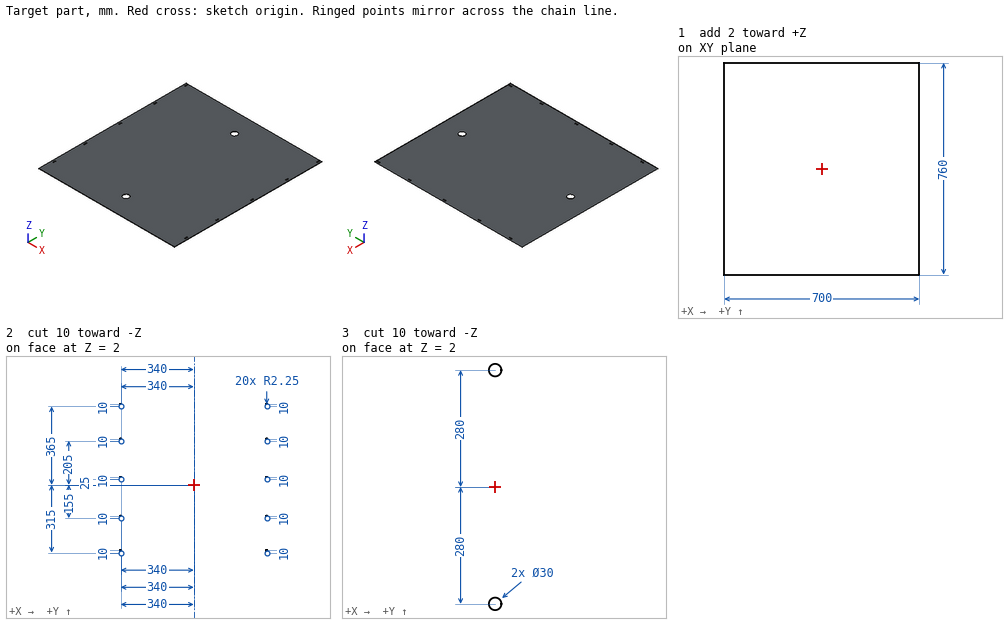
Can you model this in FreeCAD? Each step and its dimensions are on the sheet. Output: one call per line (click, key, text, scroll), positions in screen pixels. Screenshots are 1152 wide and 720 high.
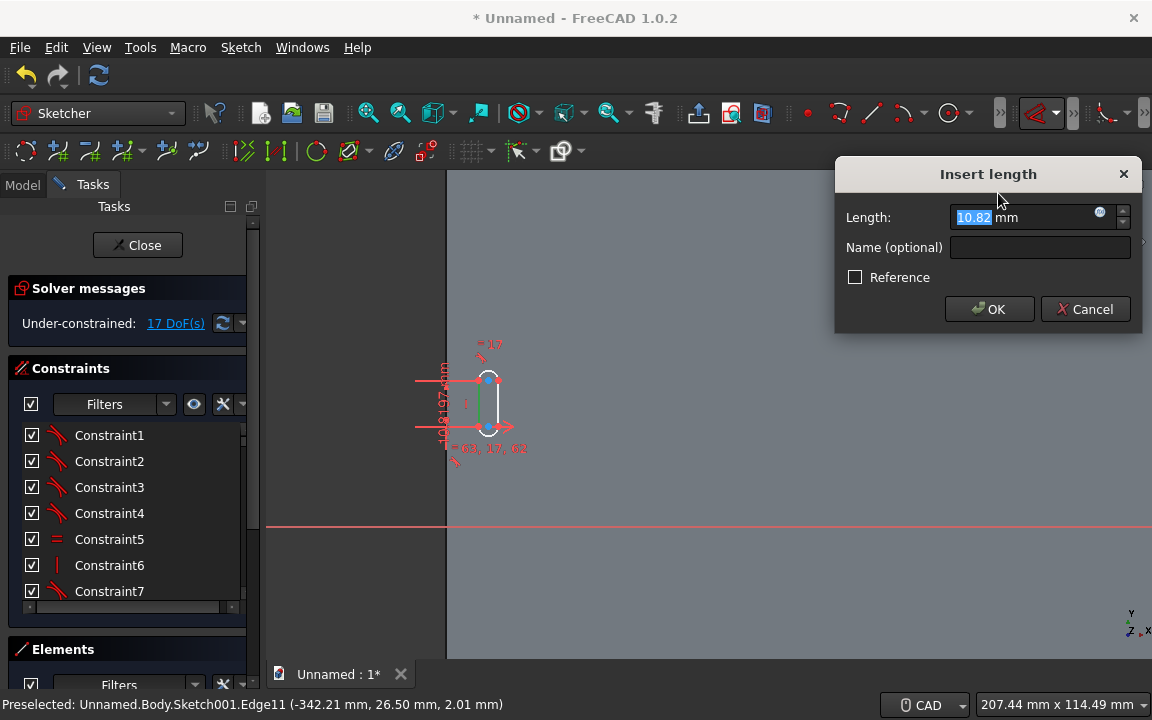
text(10)
key(Return)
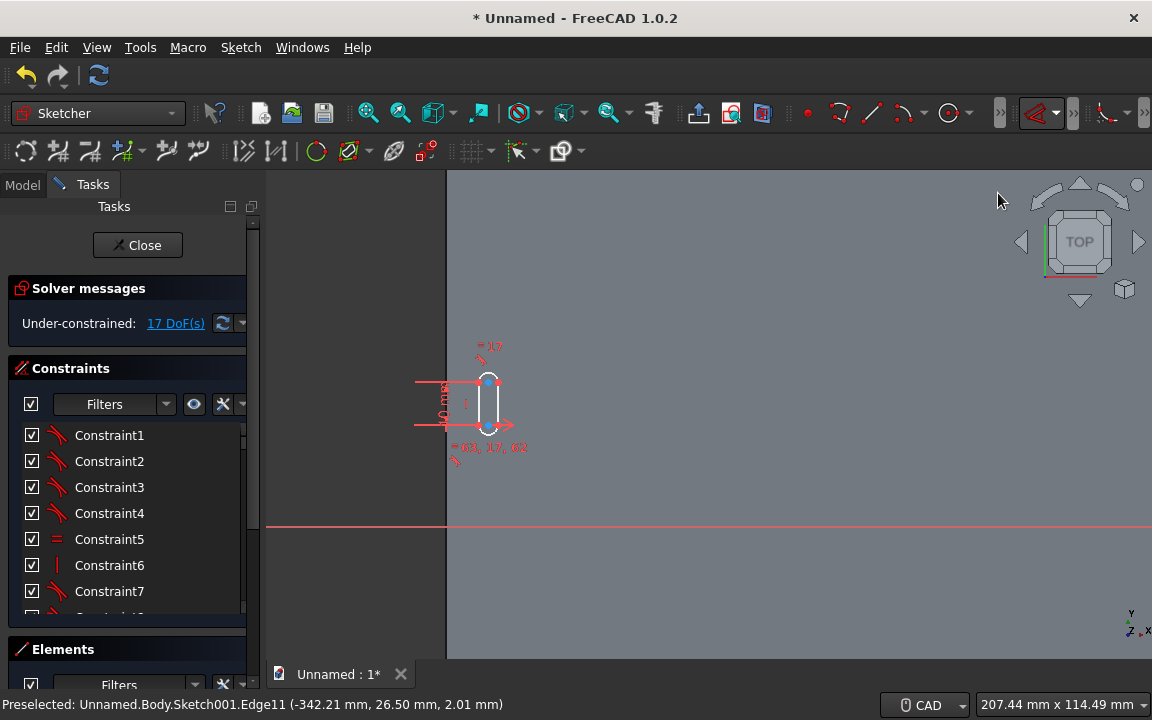
scroll(479, 416, down, 11)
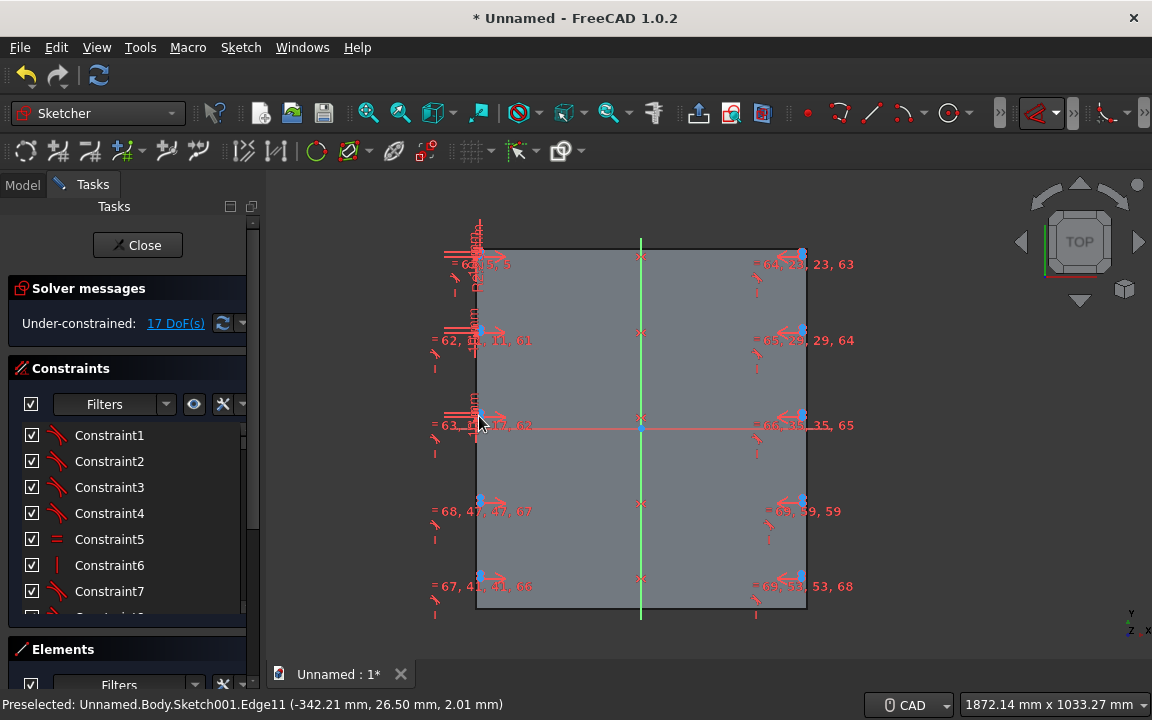
scroll(801, 255, up, 11)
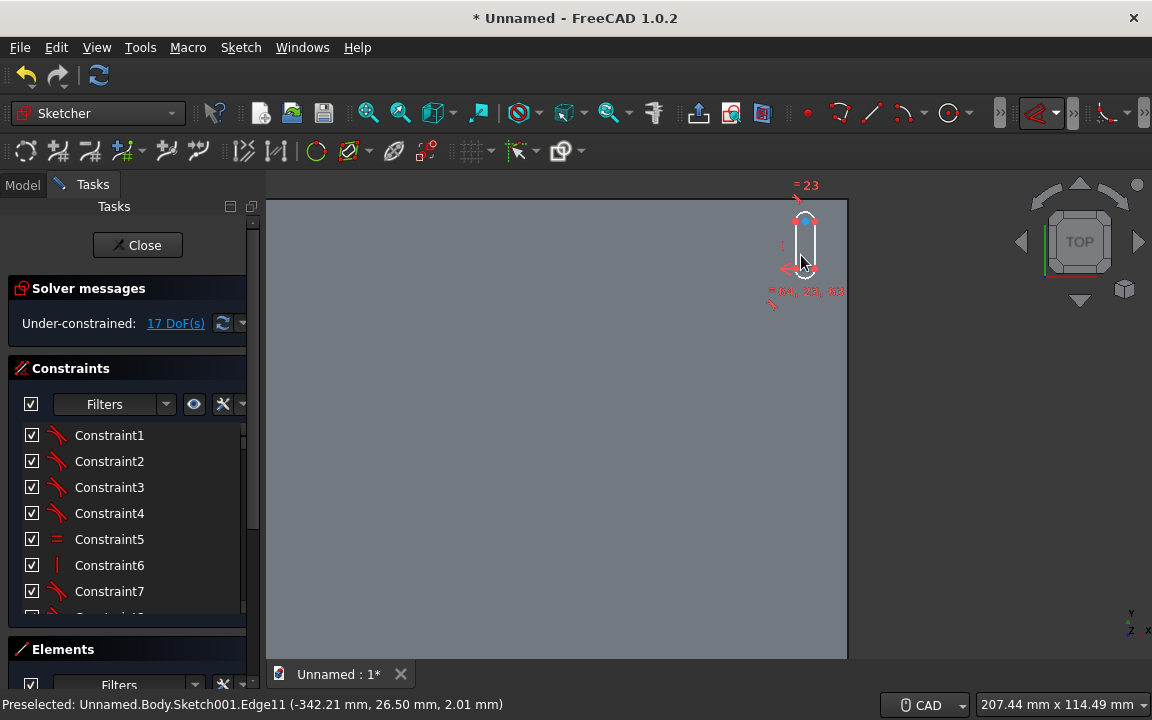
click(796, 255)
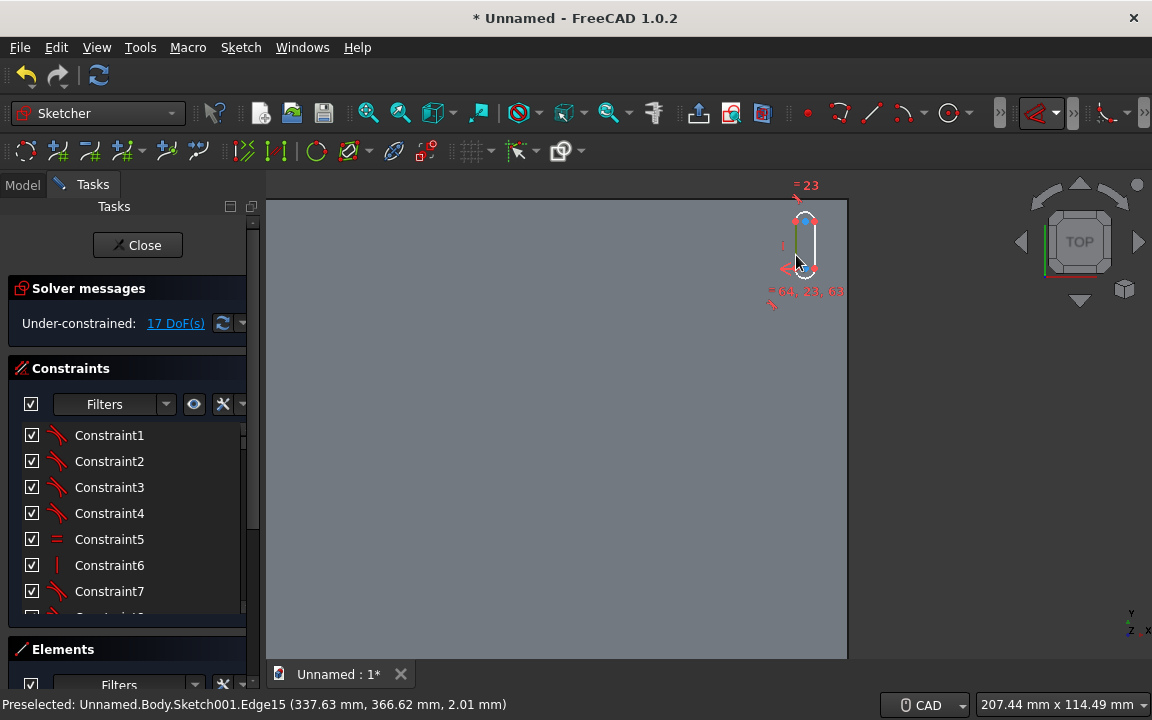
click(1058, 114)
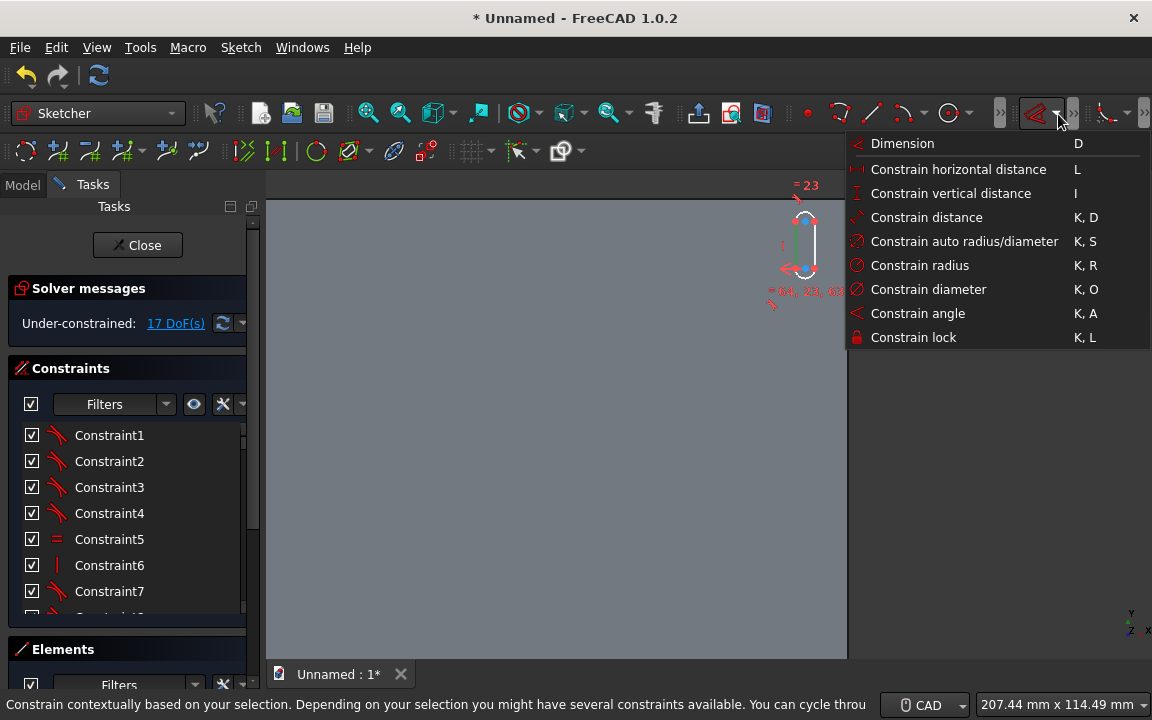
click(998, 193)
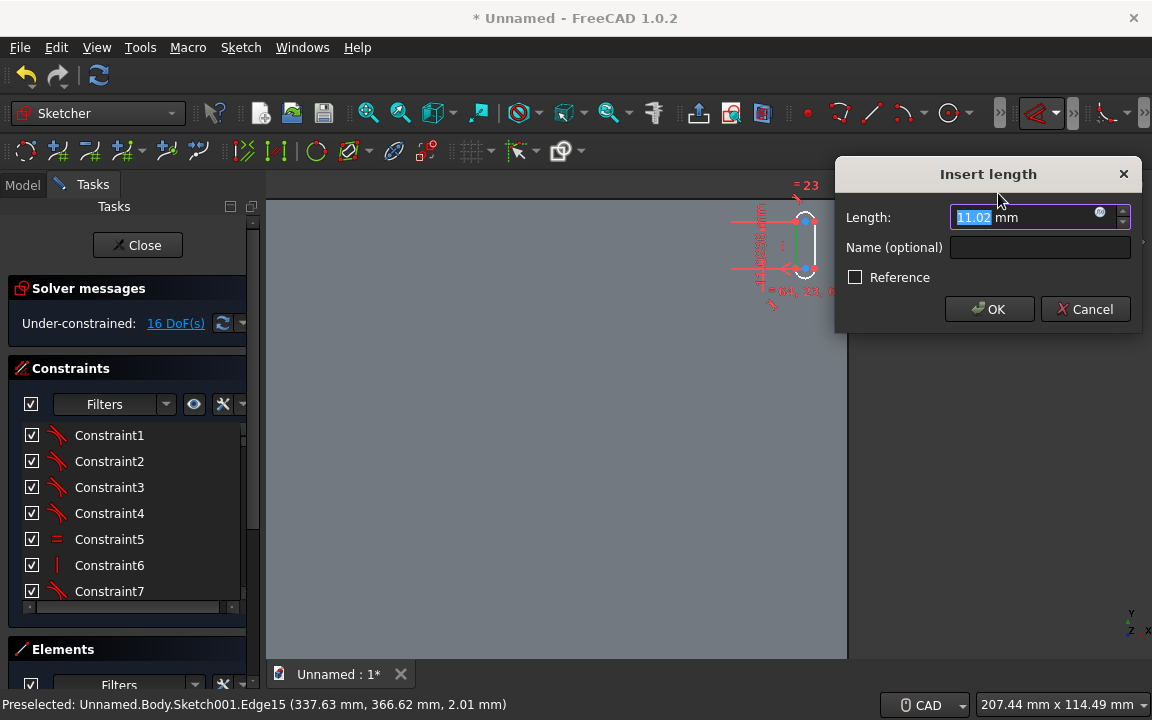
text(10)
key(Return)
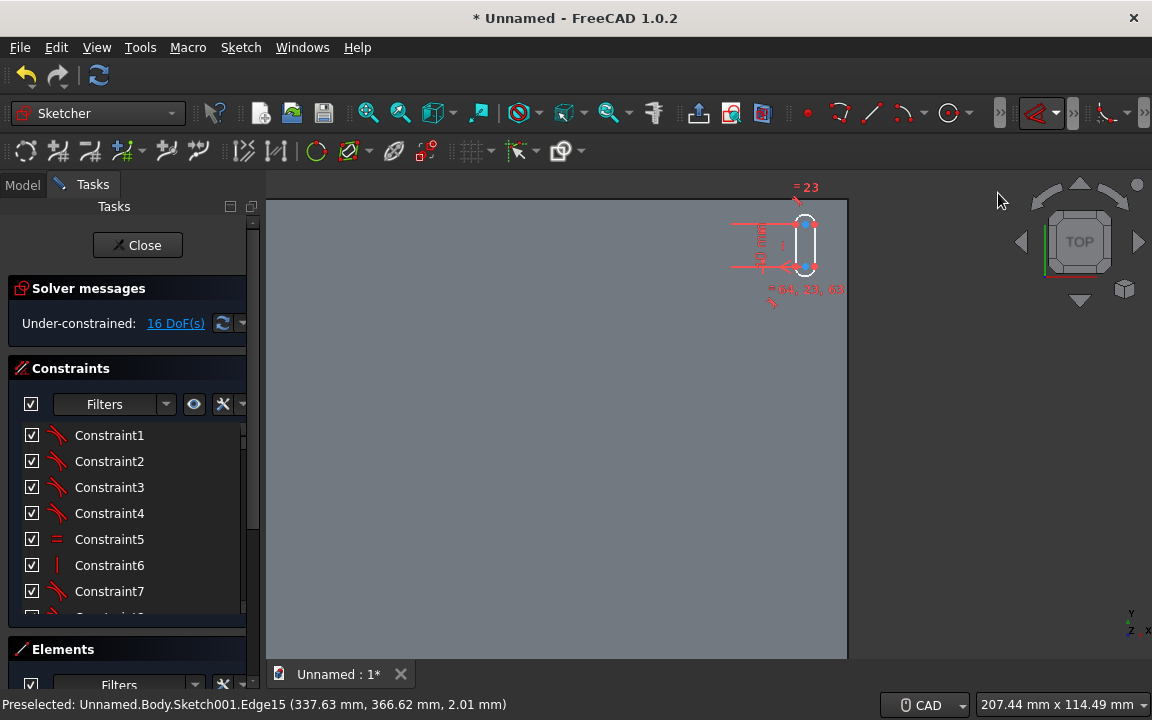
scroll(801, 255, down, 11)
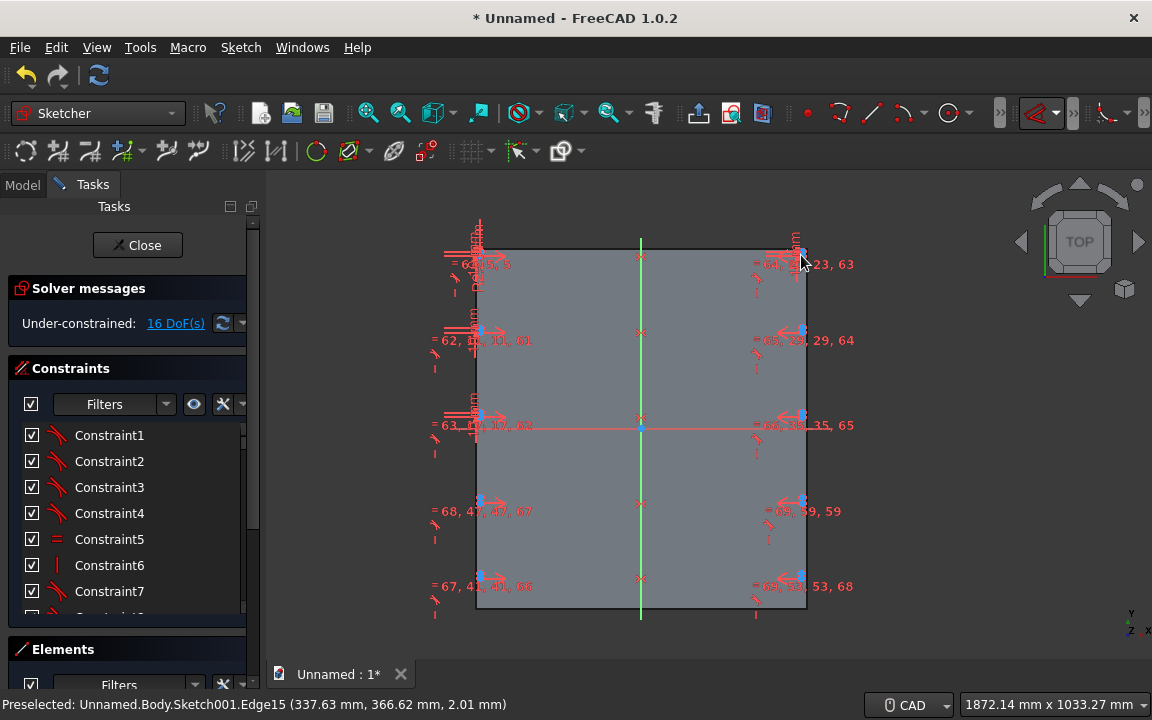
scroll(801, 331, up, 11)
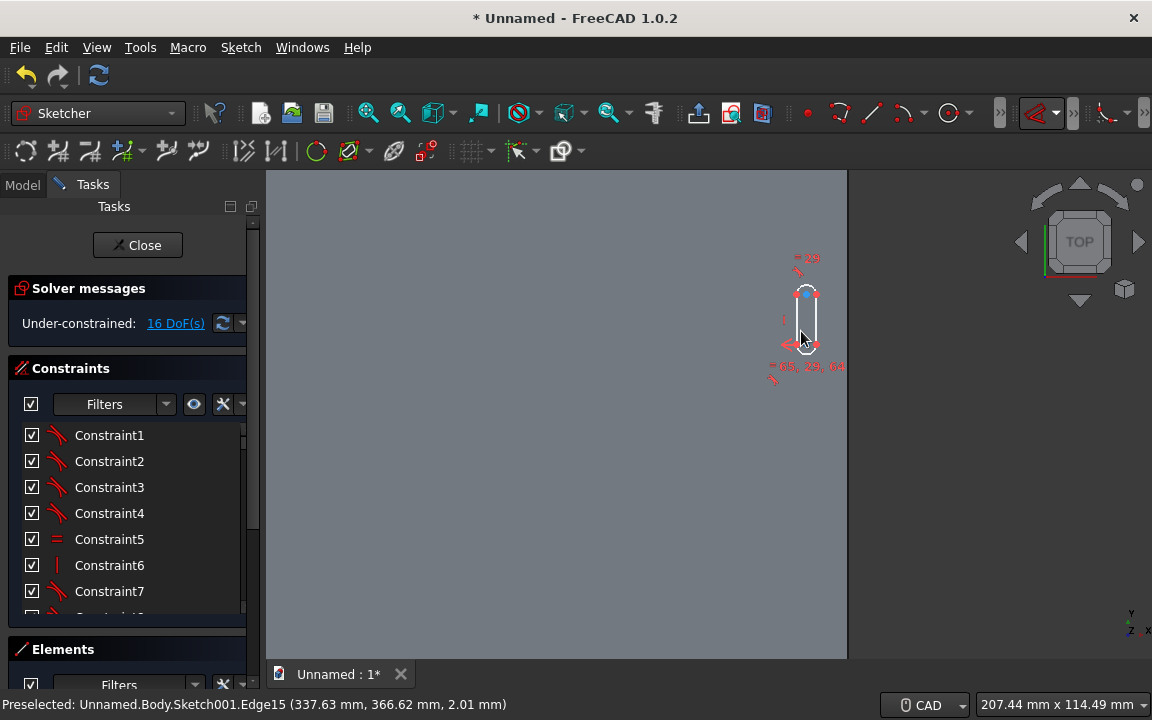
click(797, 330)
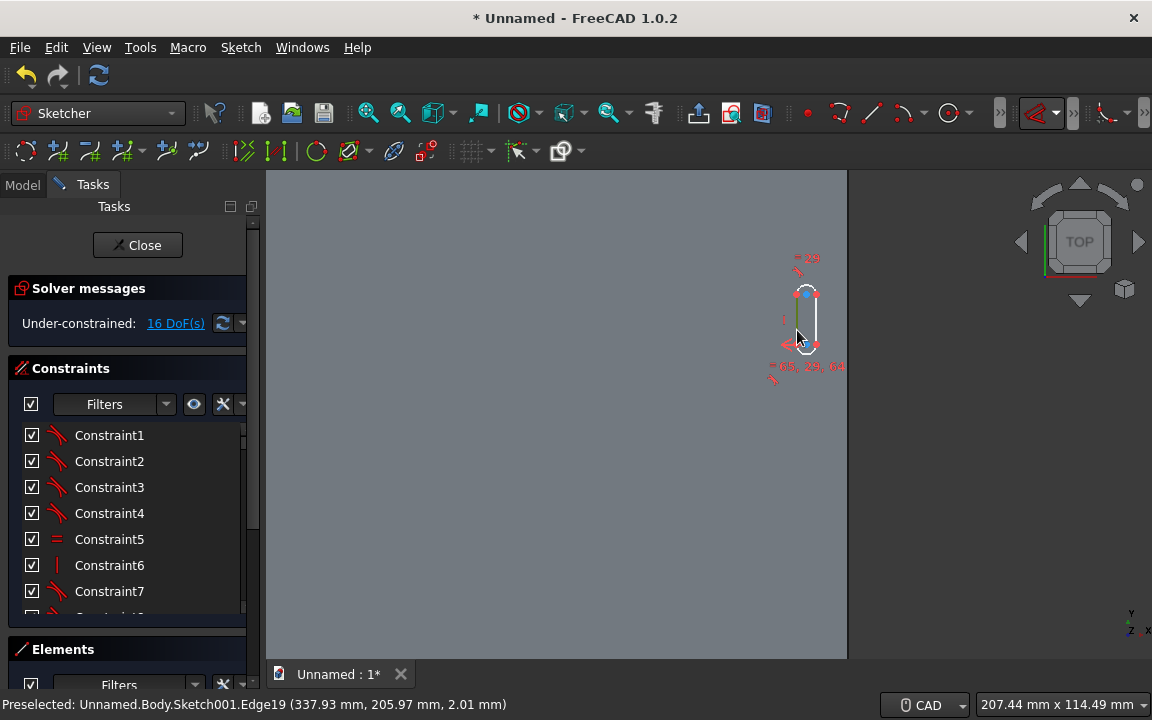
key(i)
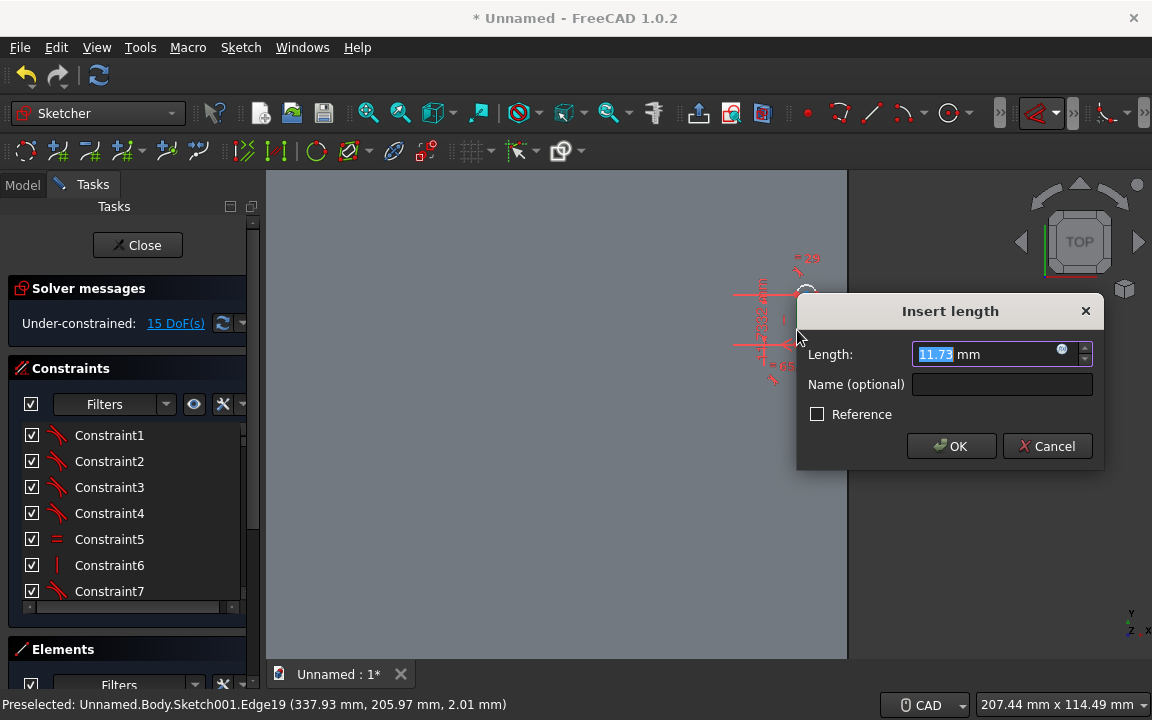
text(10)
key(Return)